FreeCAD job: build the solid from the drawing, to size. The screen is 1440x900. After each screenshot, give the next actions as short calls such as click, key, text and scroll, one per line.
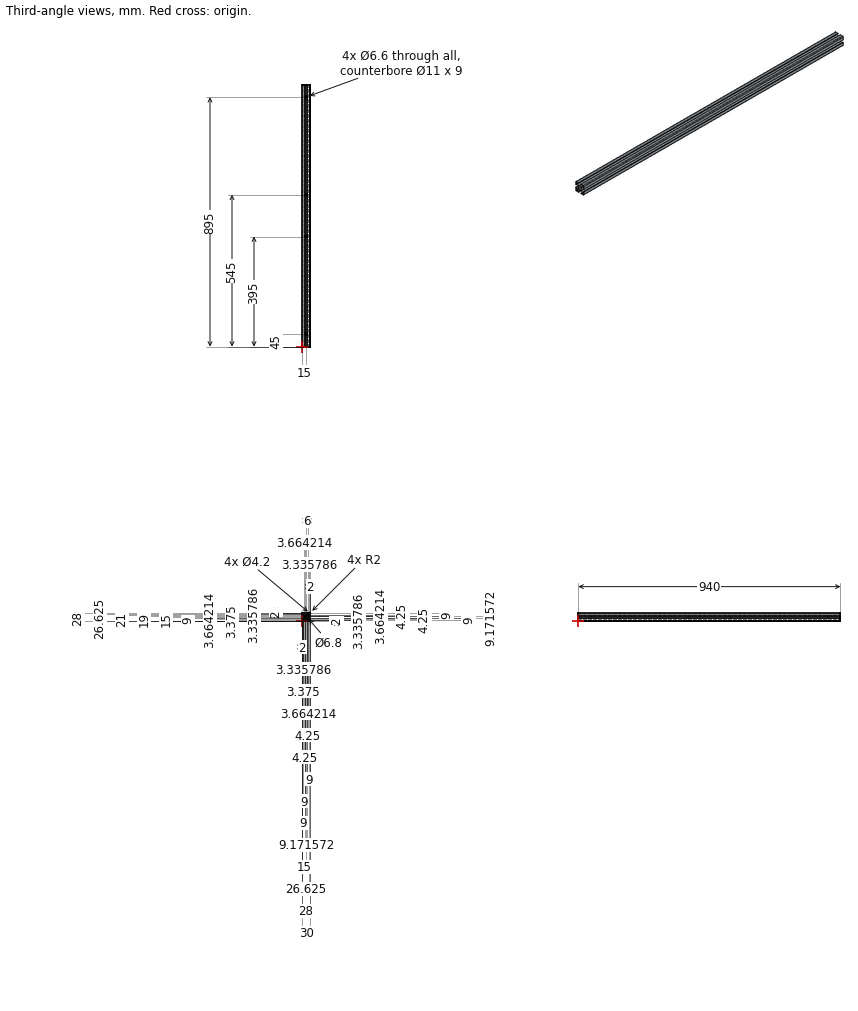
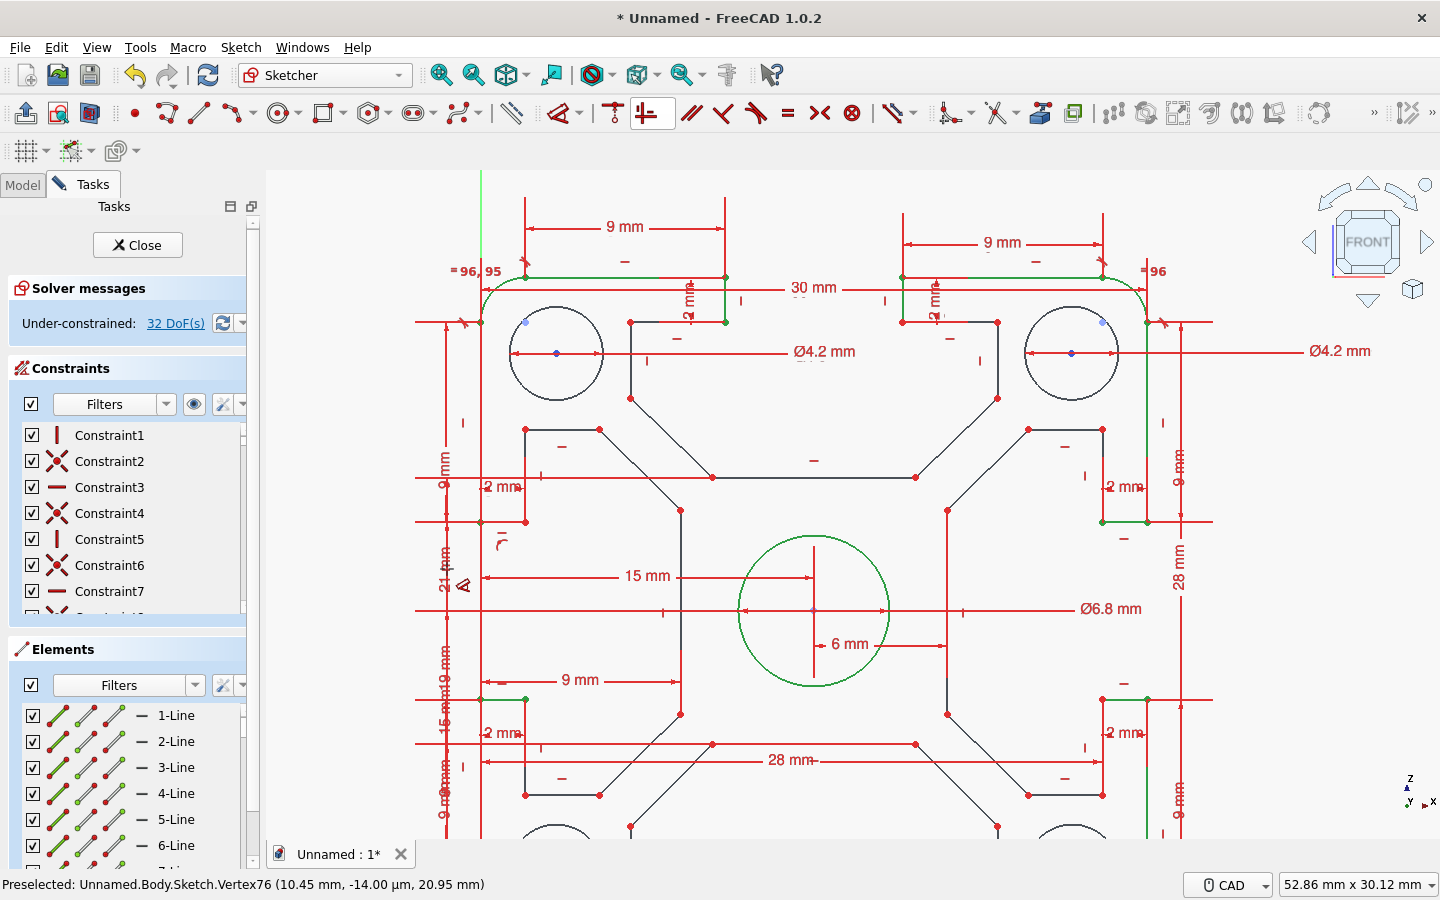
click(1103, 494)
click(1069, 455)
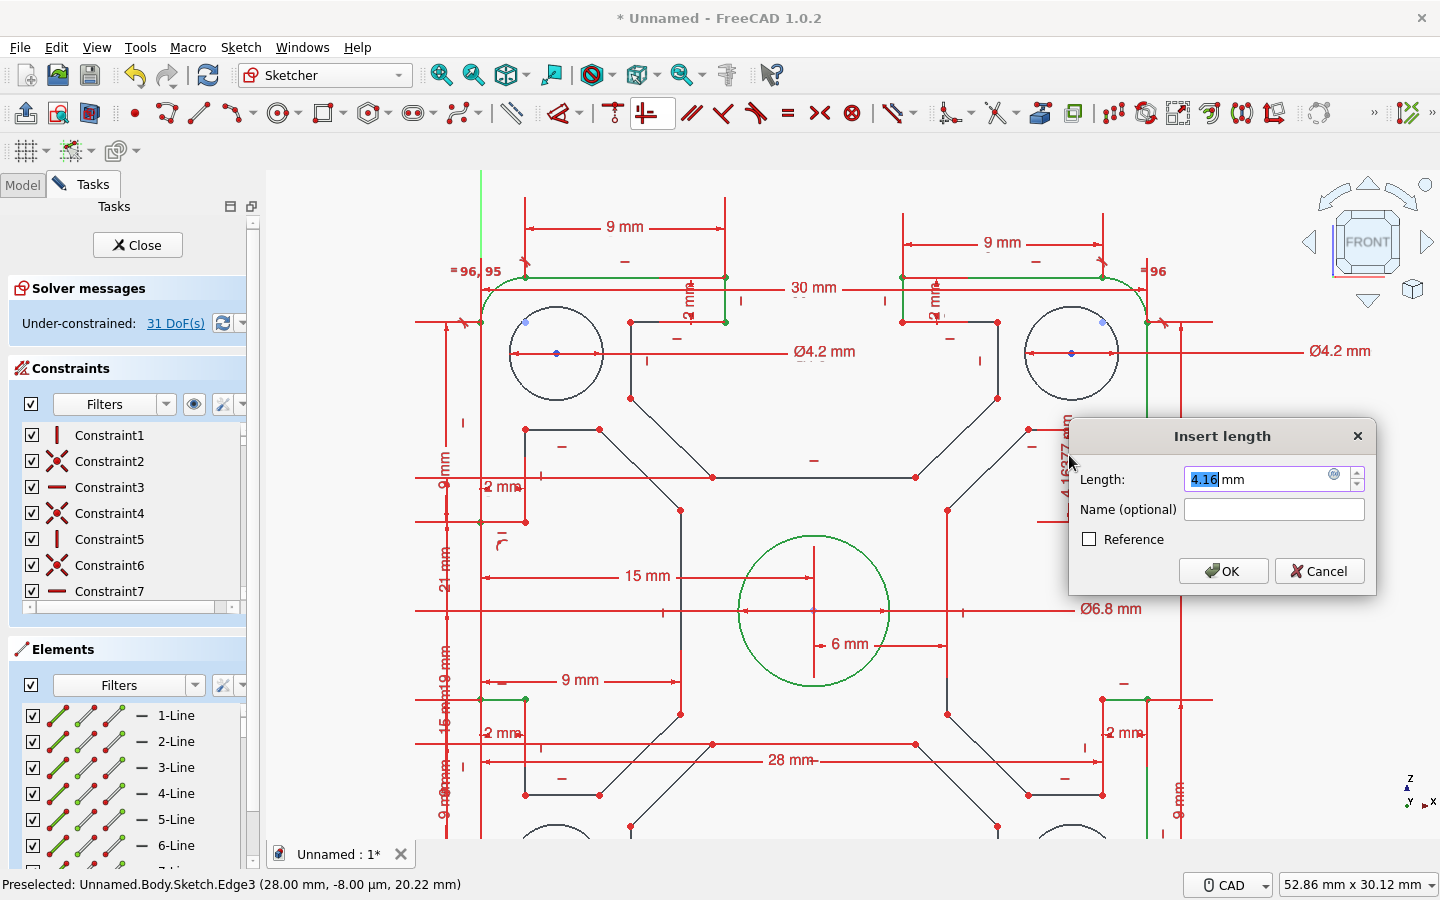
text(4.25)
key(Return)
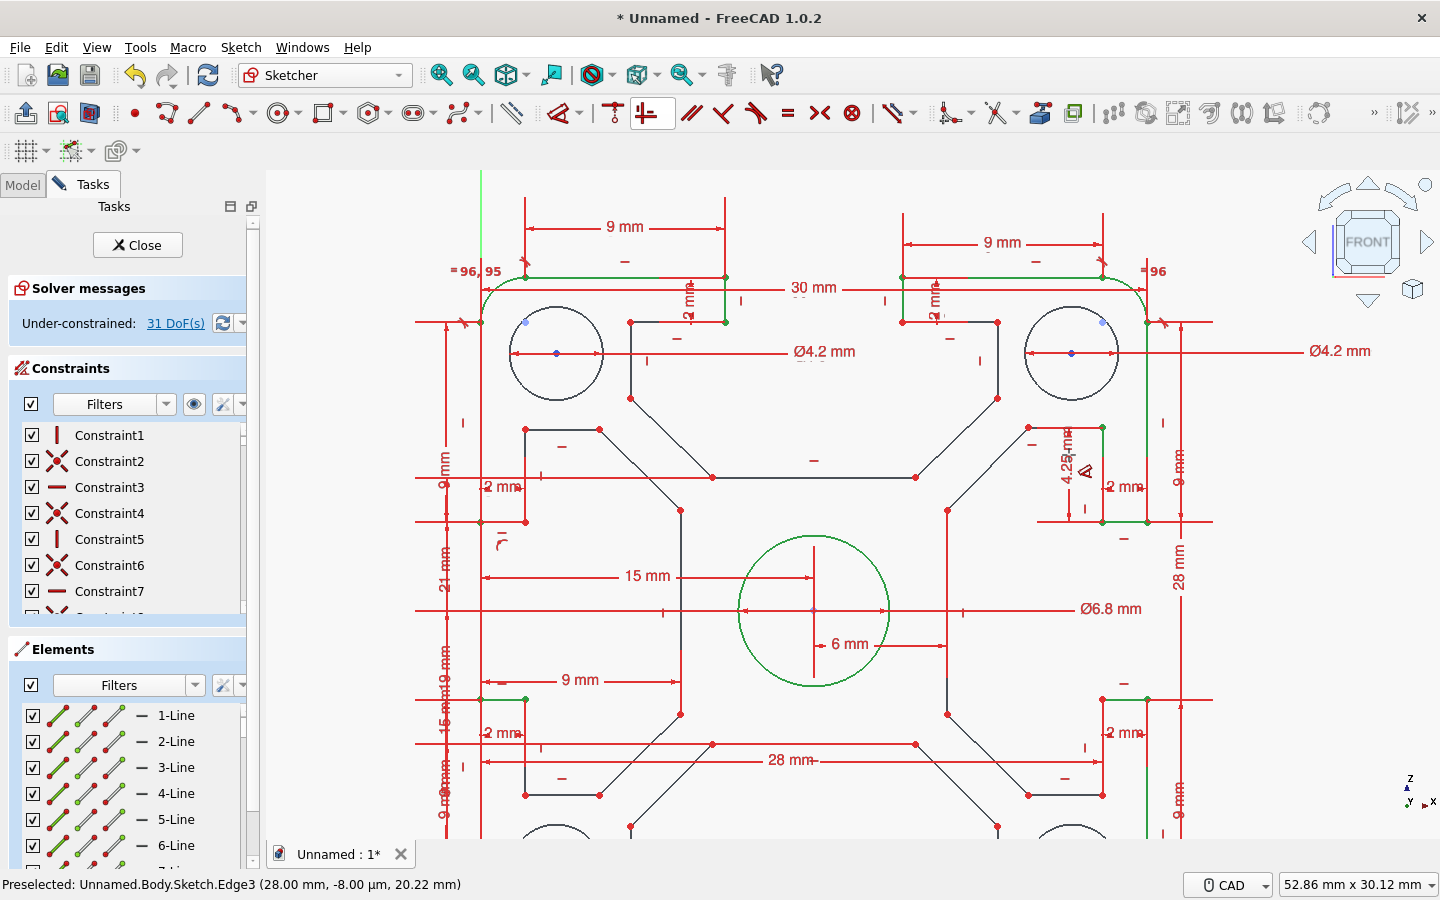
click(1103, 767)
click(1069, 769)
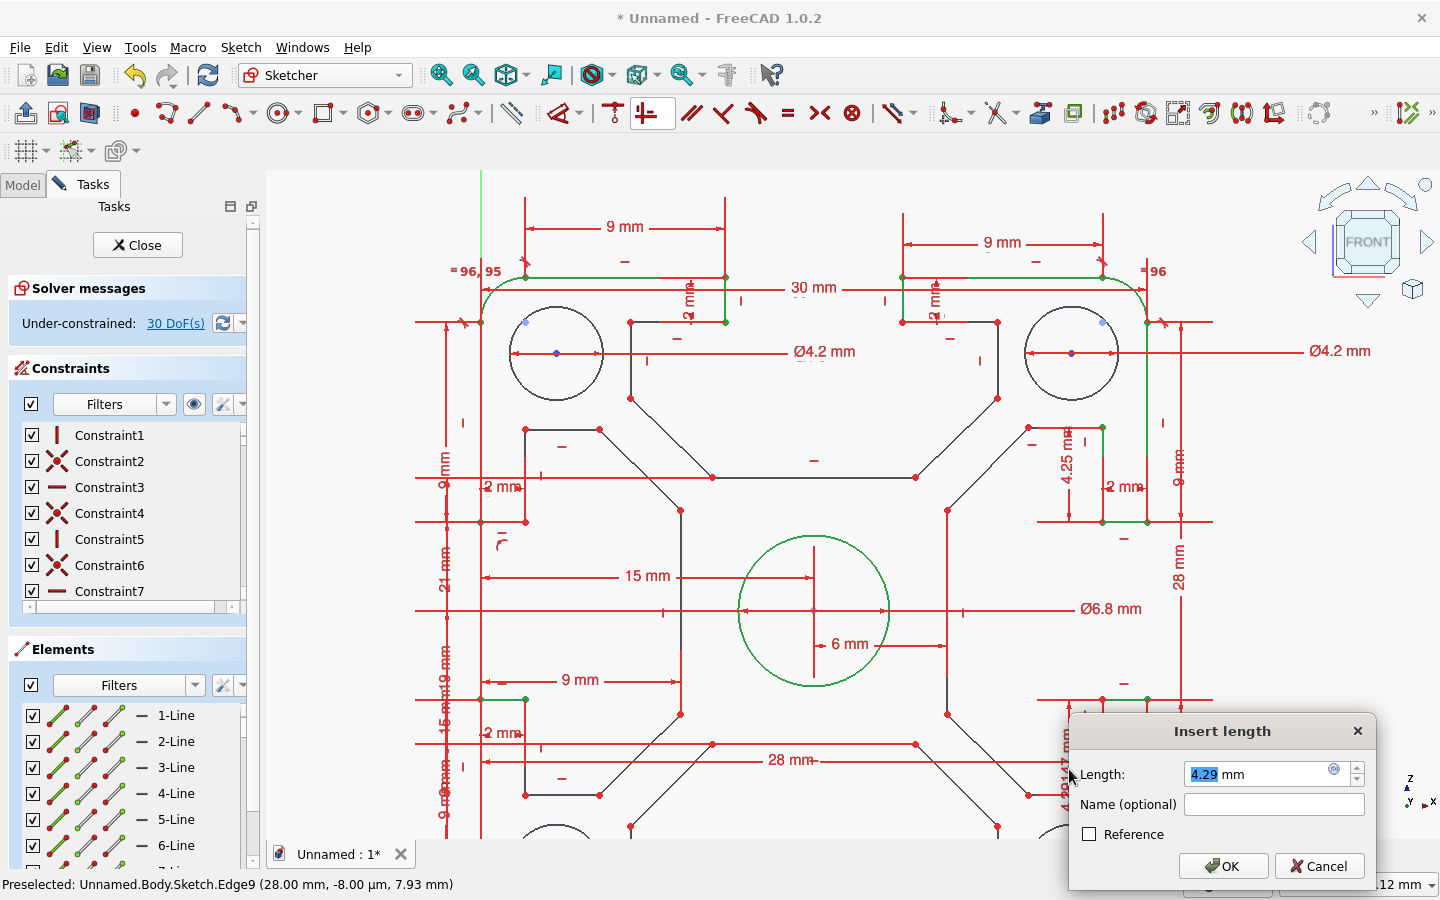
text(4.25)
key(Return)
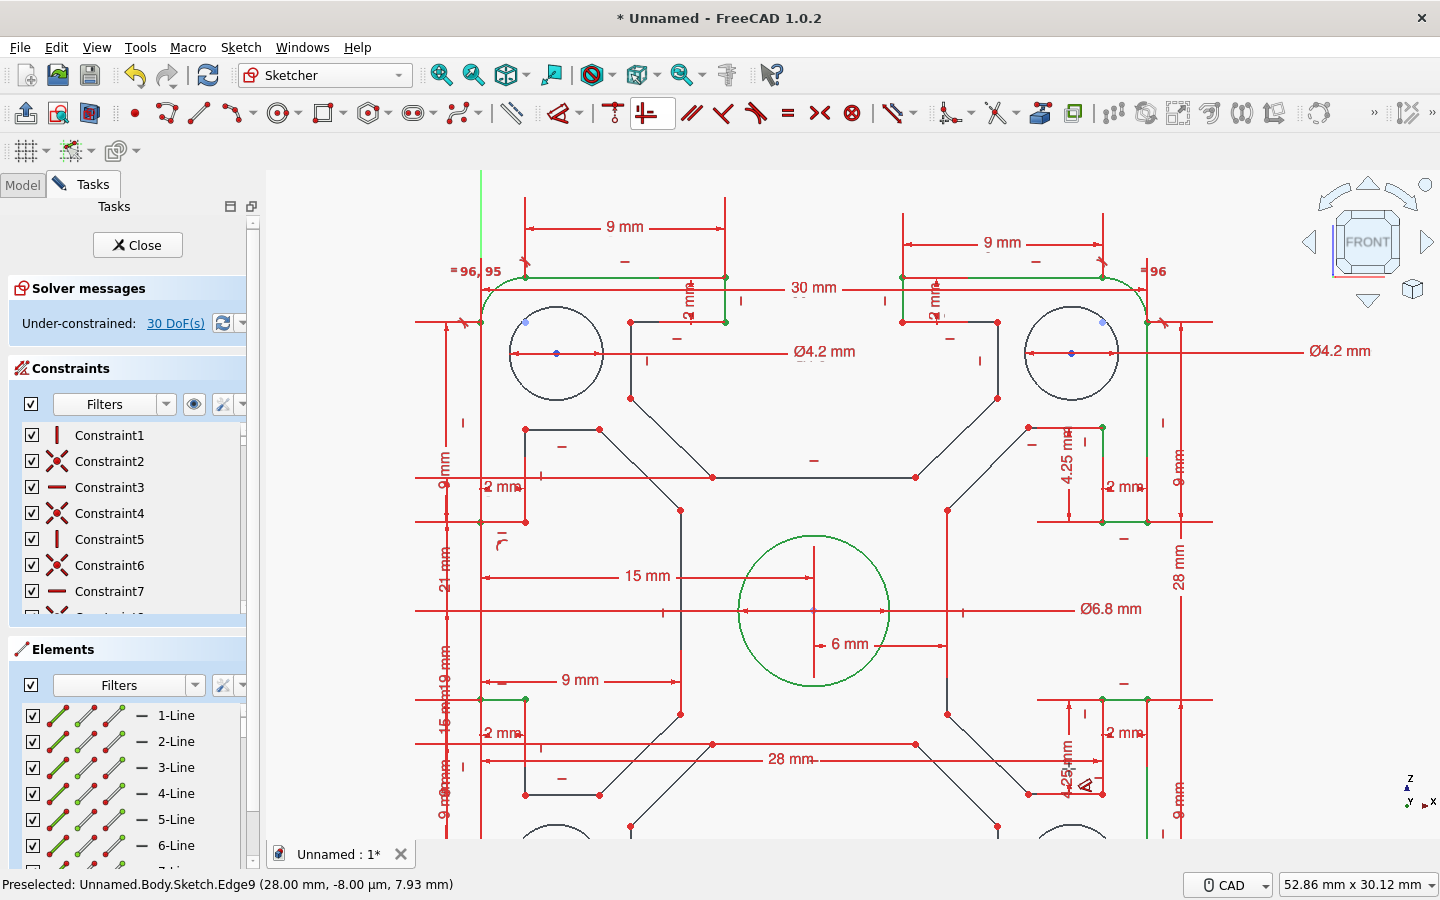
scroll(725, 288, down, 2)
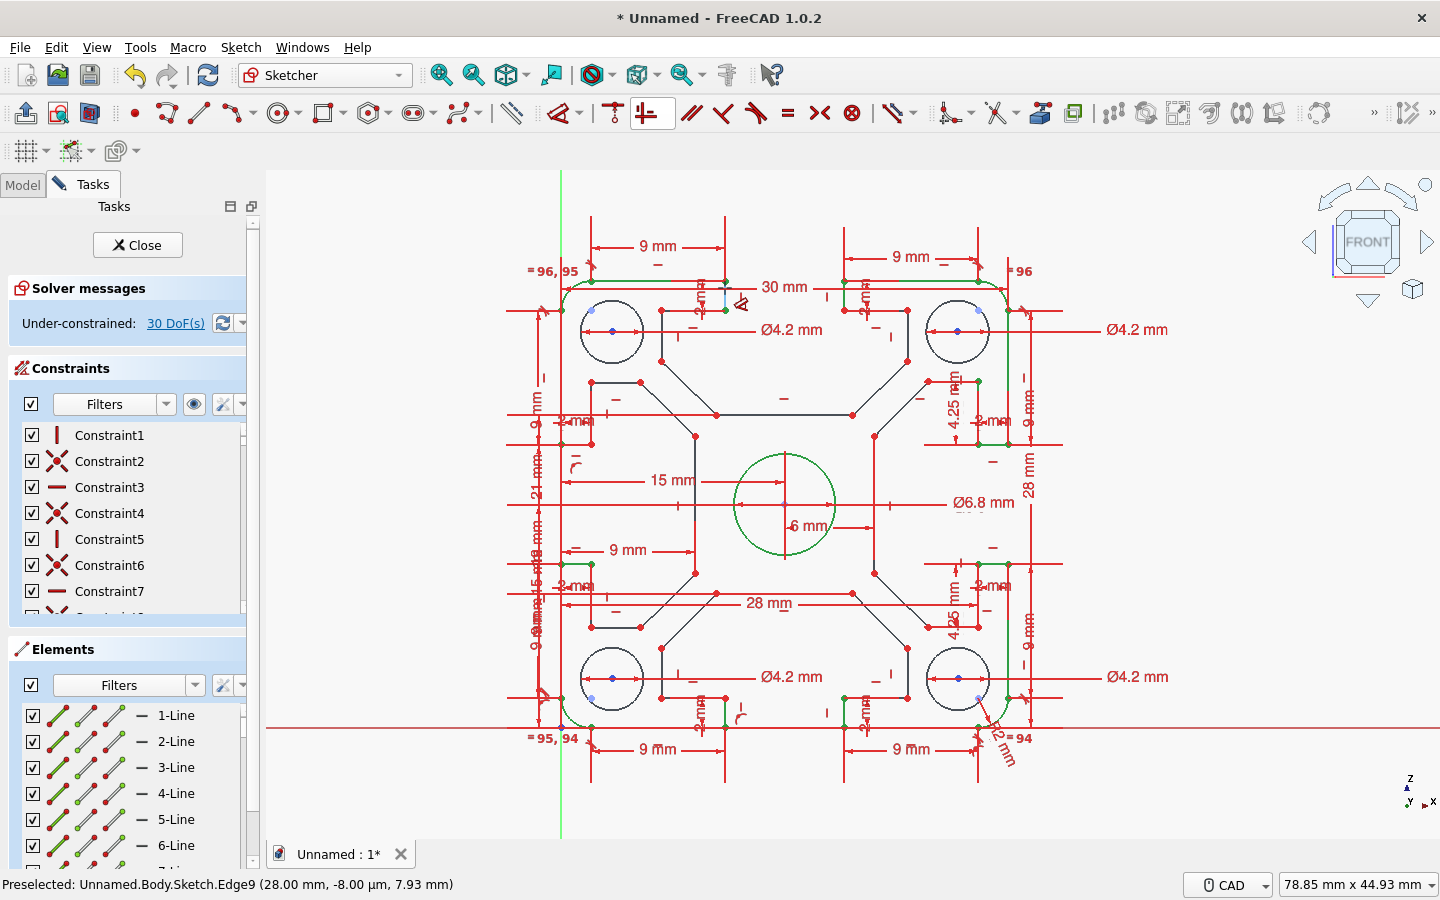
click(863, 698)
click(876, 664)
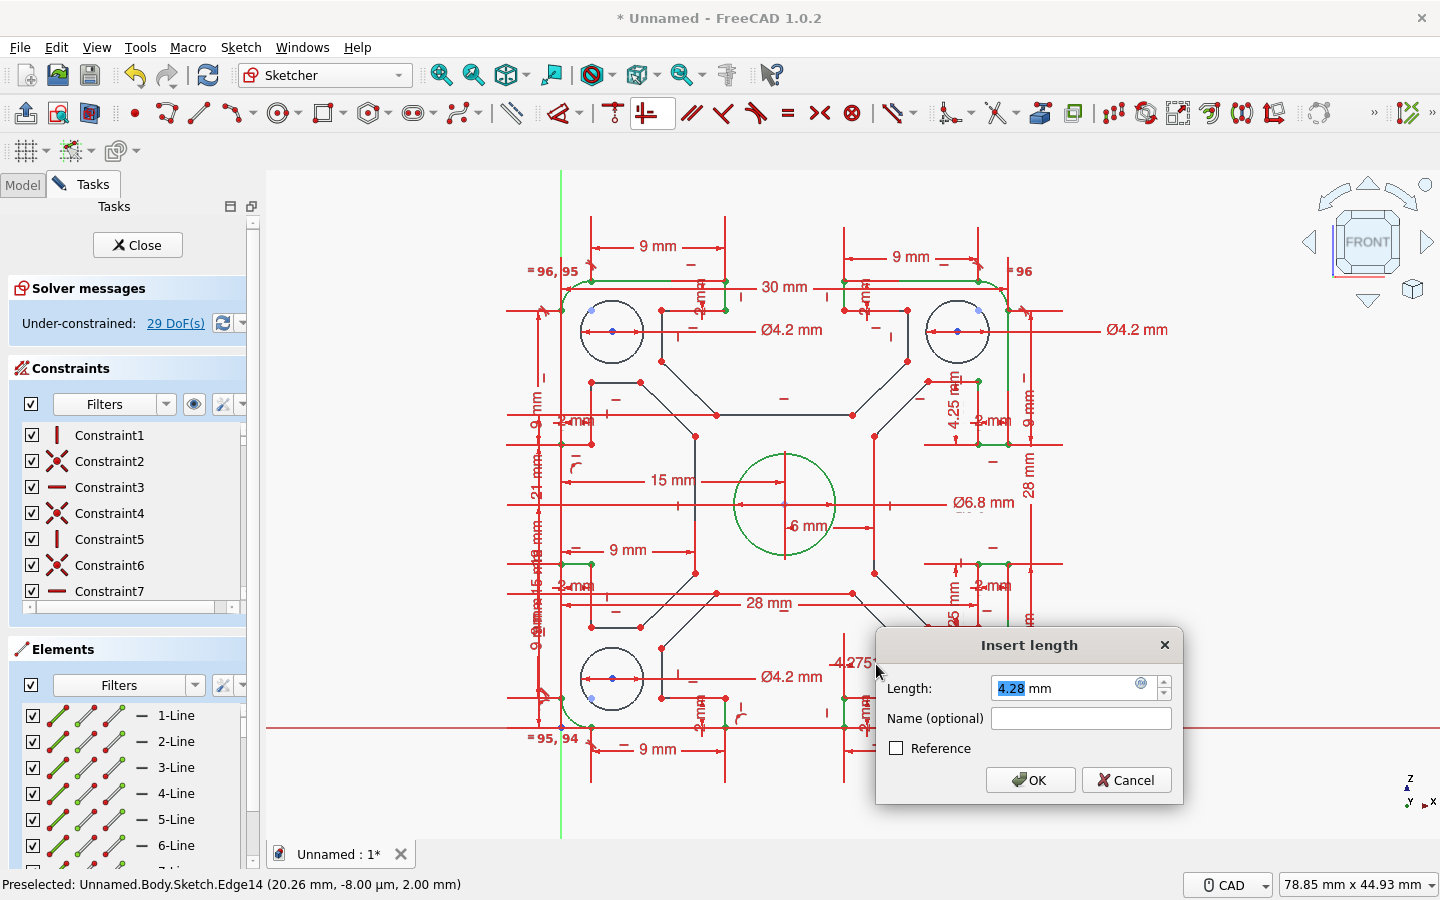
text(4.25)
key(Return)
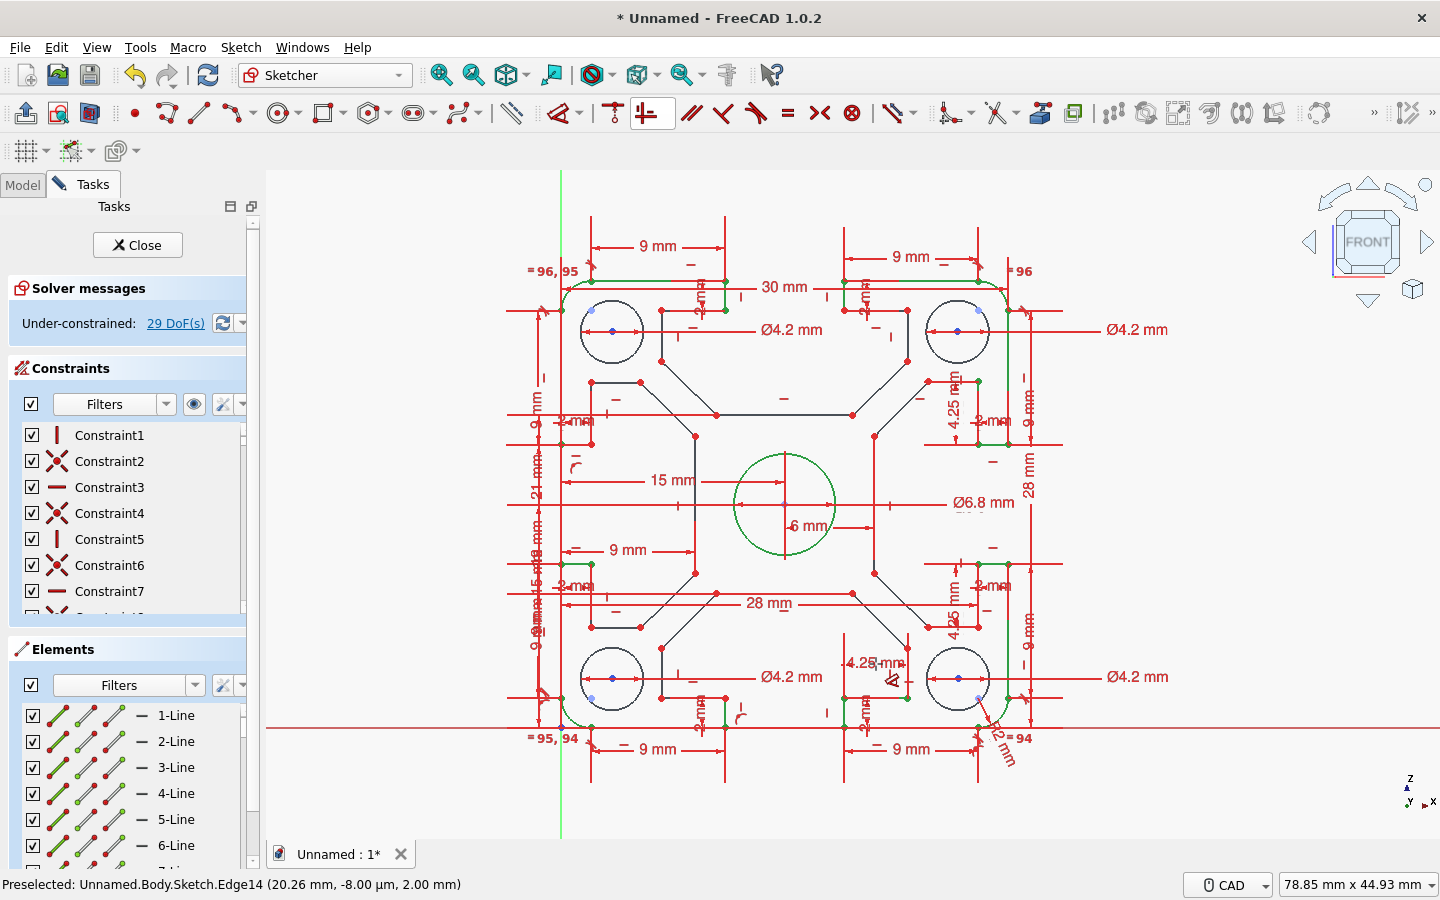
click(681, 698)
click(694, 664)